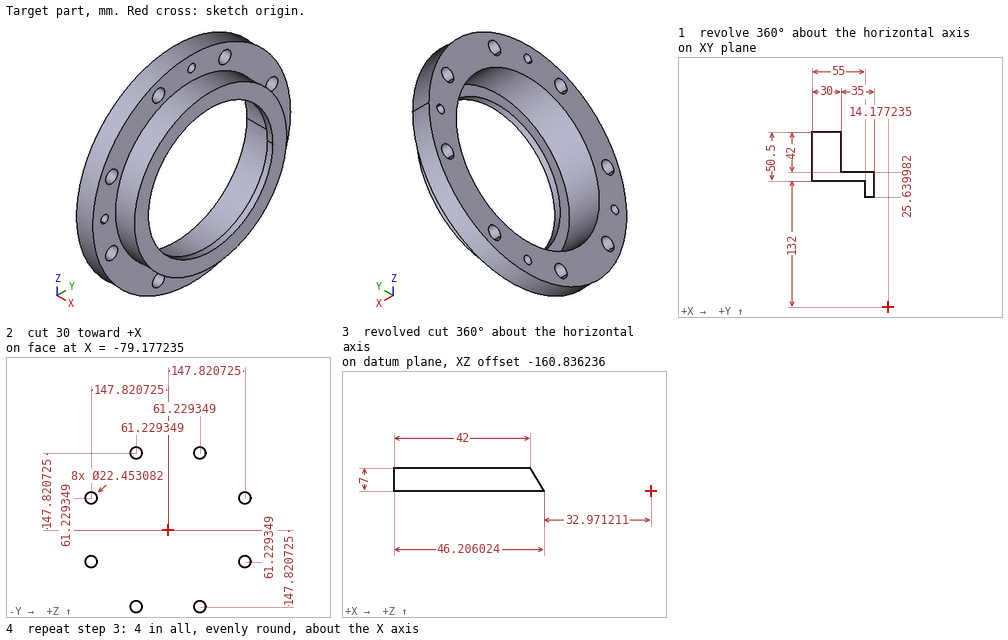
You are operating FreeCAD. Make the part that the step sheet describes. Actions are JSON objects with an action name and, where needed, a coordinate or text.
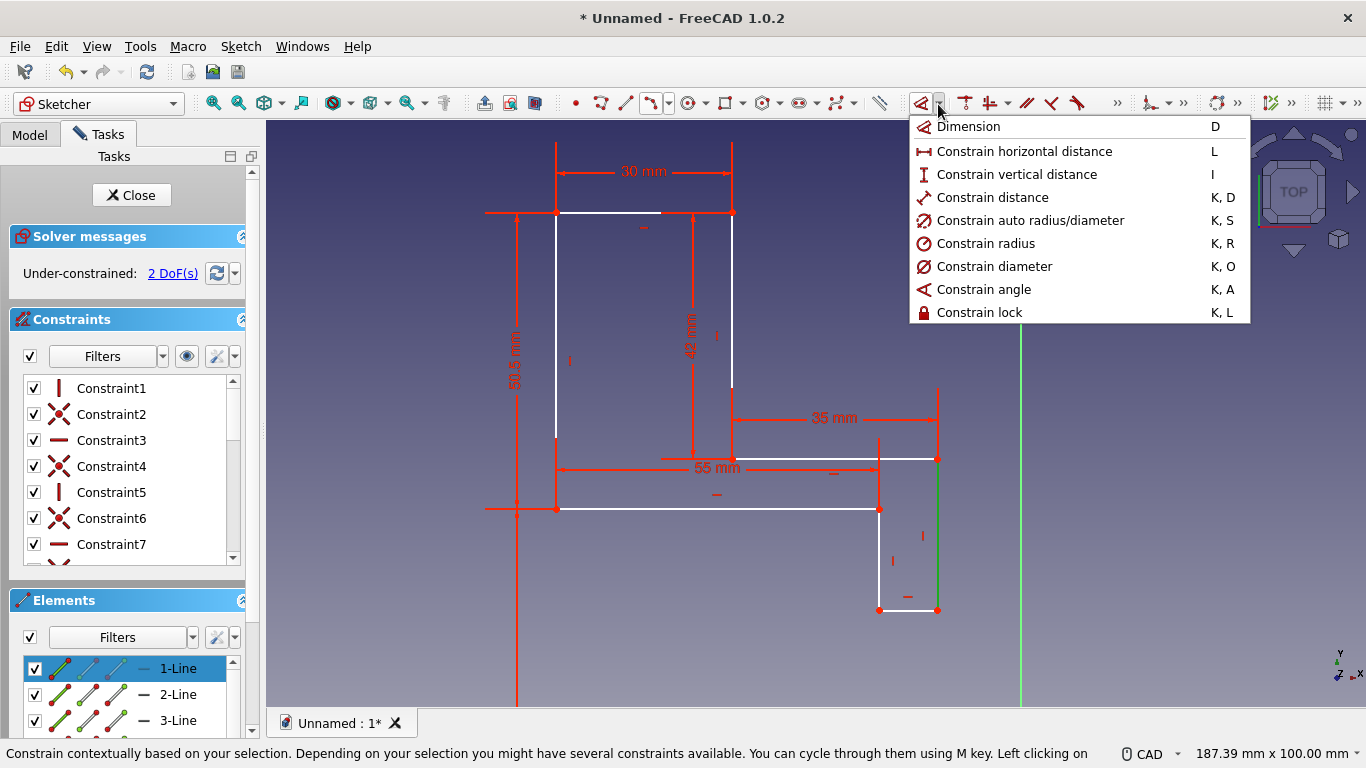
{"action": "left_click", "coordinate": [1080, 174]}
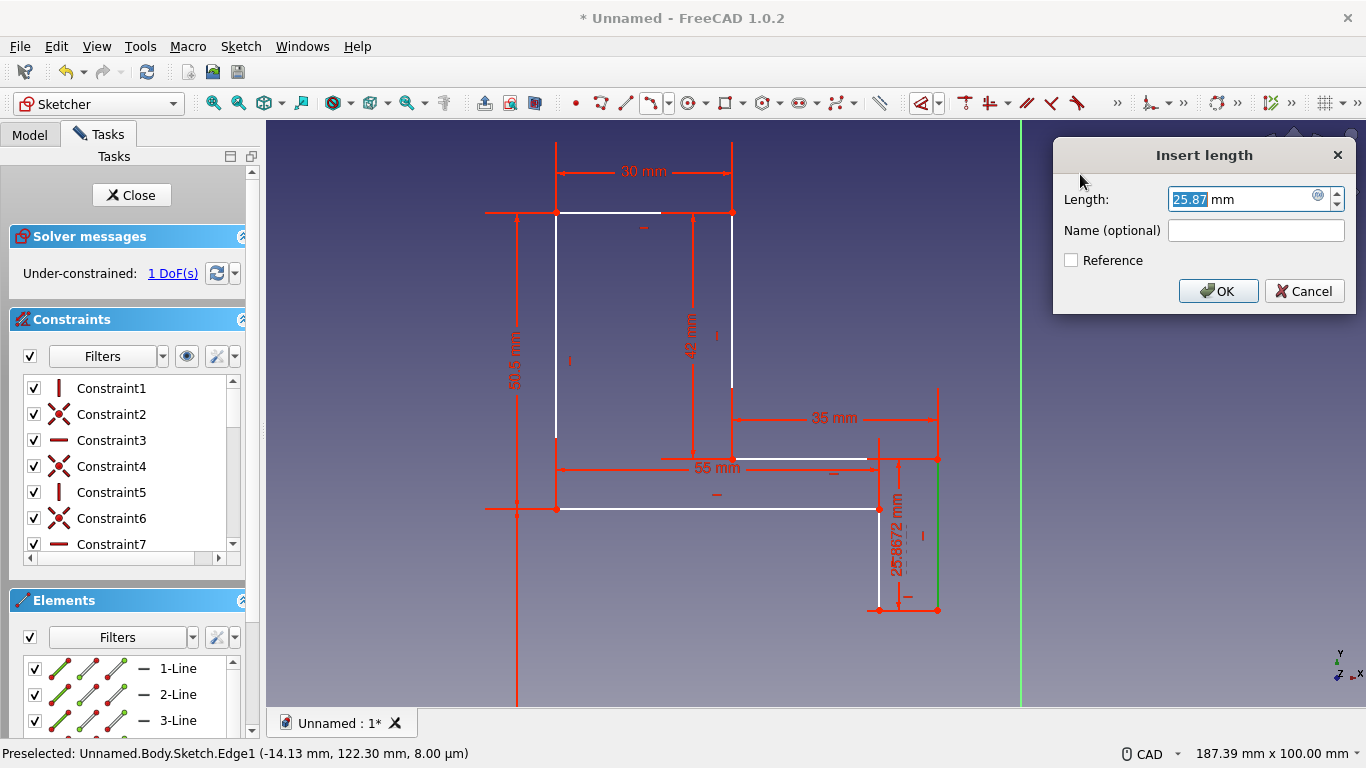
{"action": "type", "text": "25.639982"}
{"action": "key", "text": "Return"}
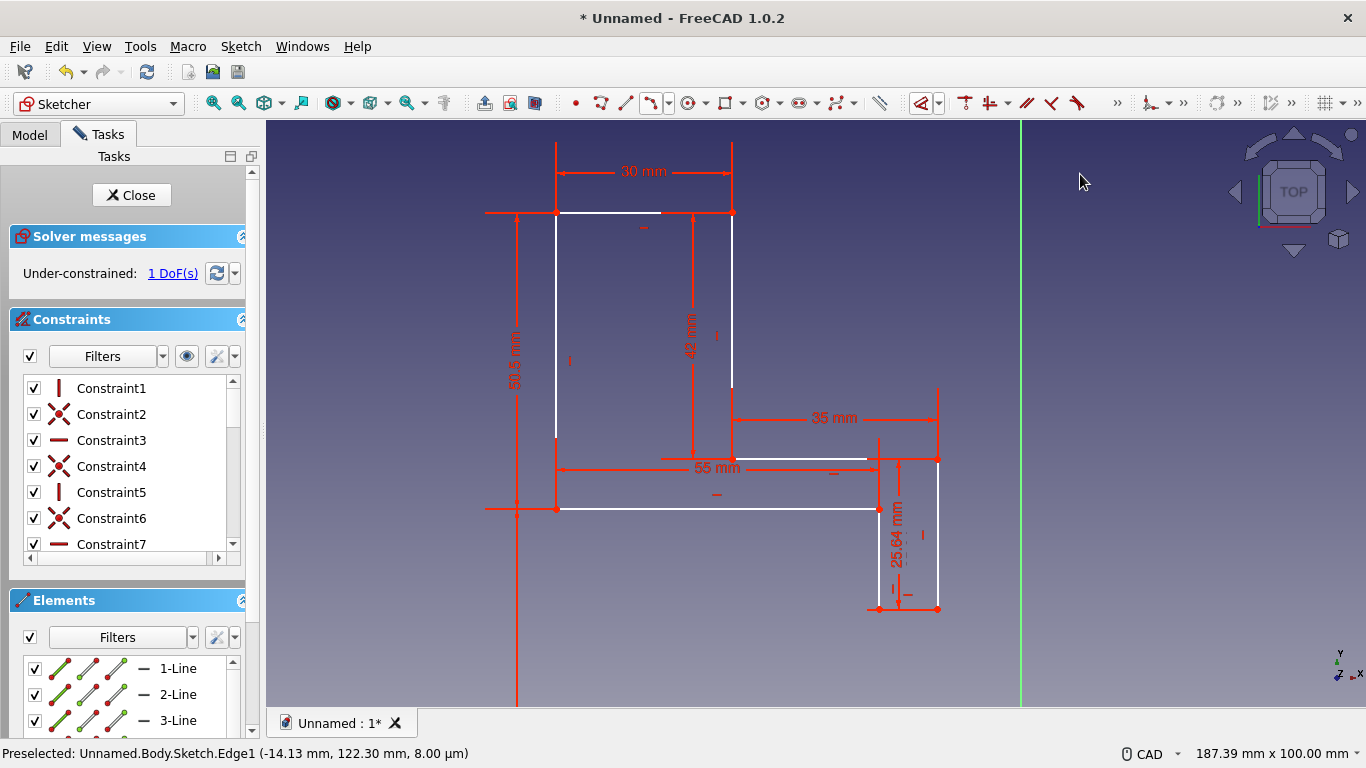
{"action": "left_click", "coordinate": [938, 610]}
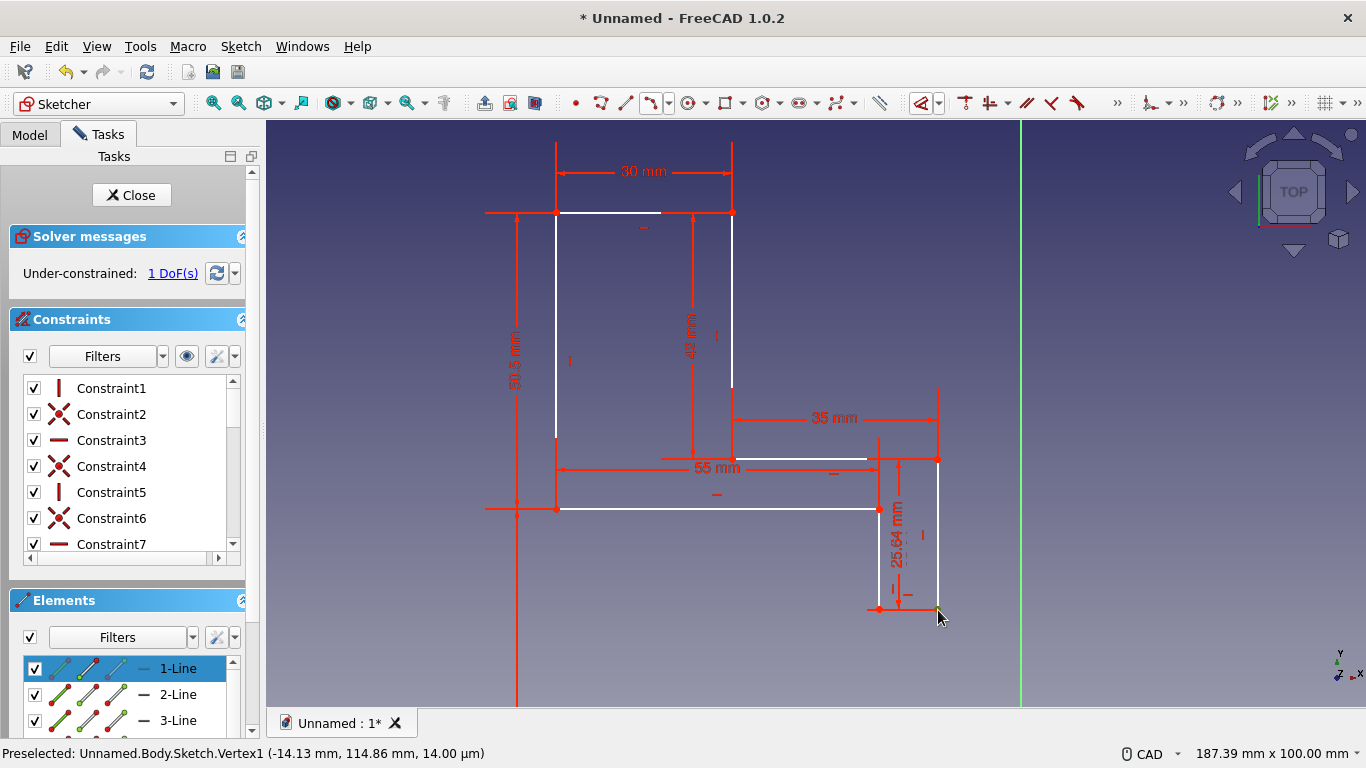
{"action": "left_click", "coordinate": [938, 104]}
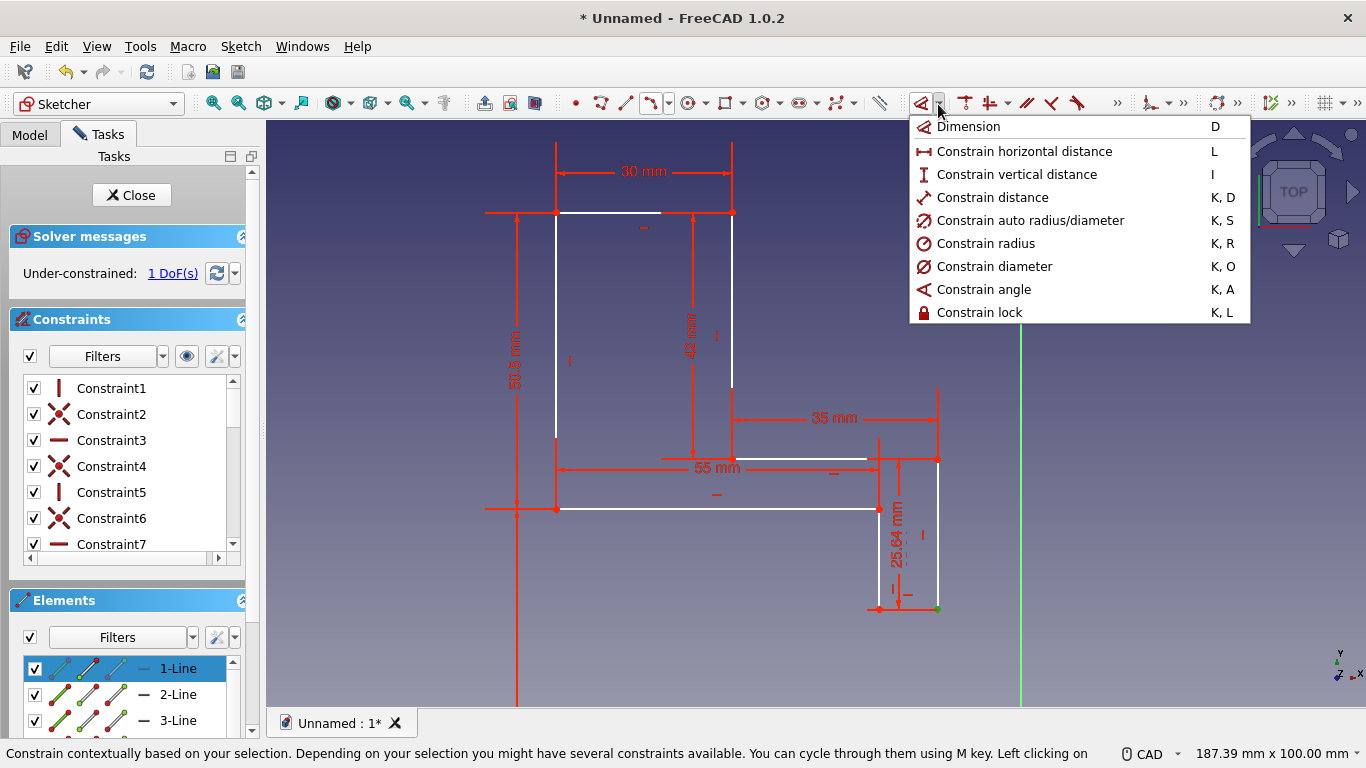
{"action": "left_click", "coordinate": [1080, 152]}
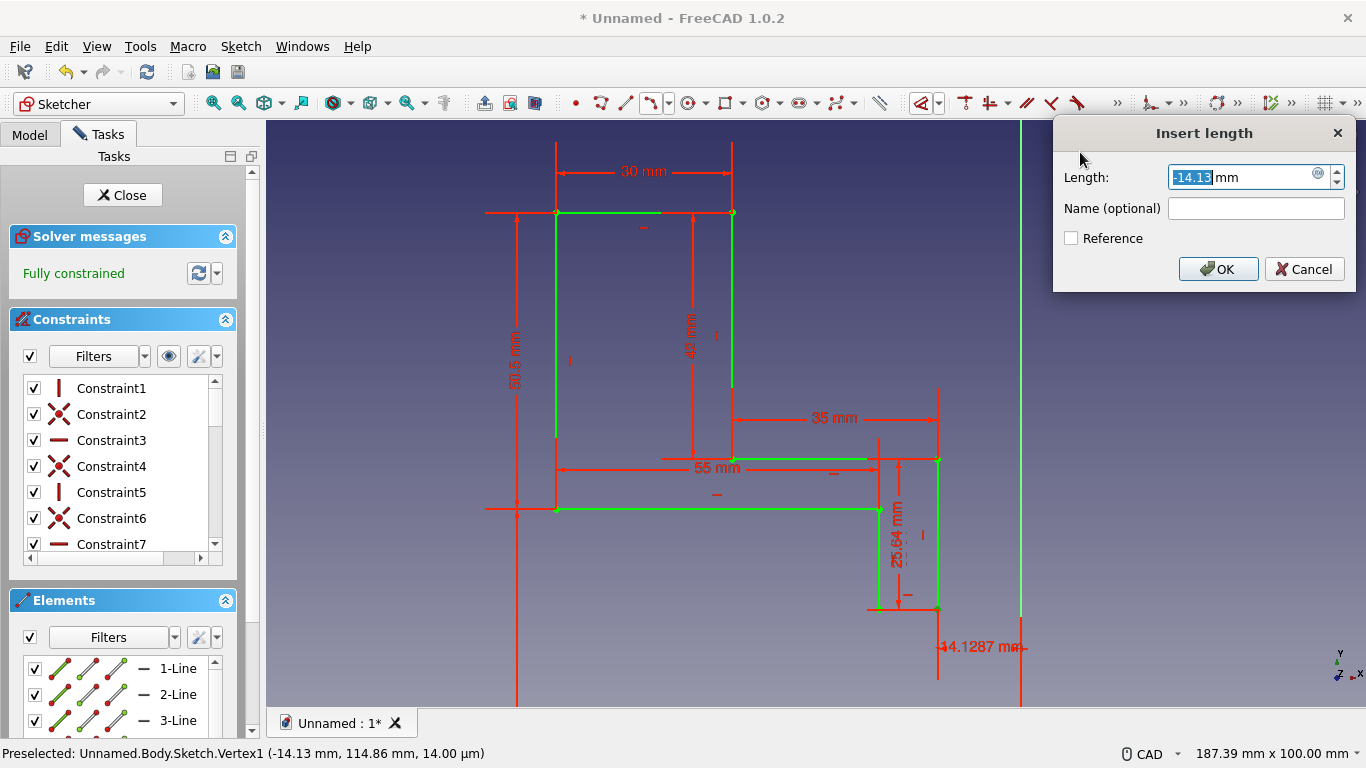
{"action": "type", "text": "-14.177235"}
{"action": "key", "text": "Return"}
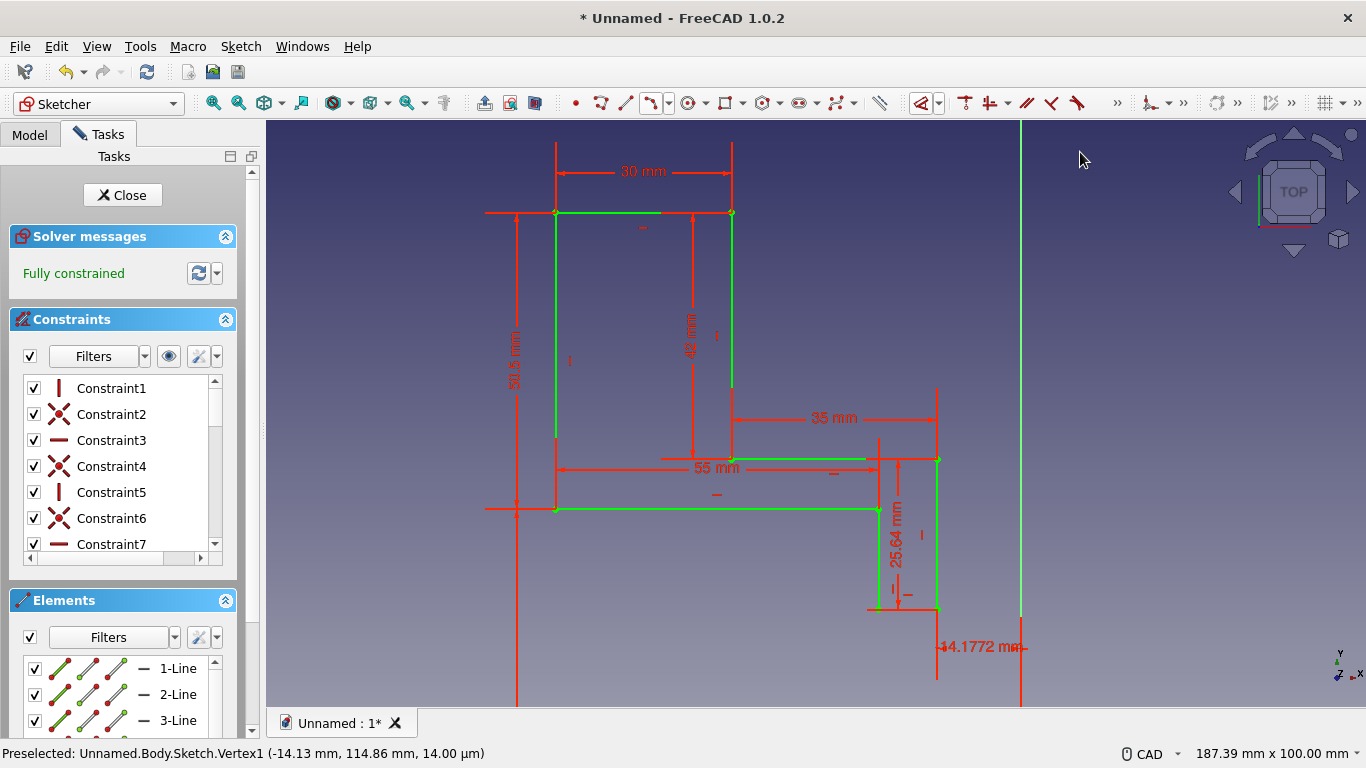
{"action": "left_click", "coordinate": [123, 195]}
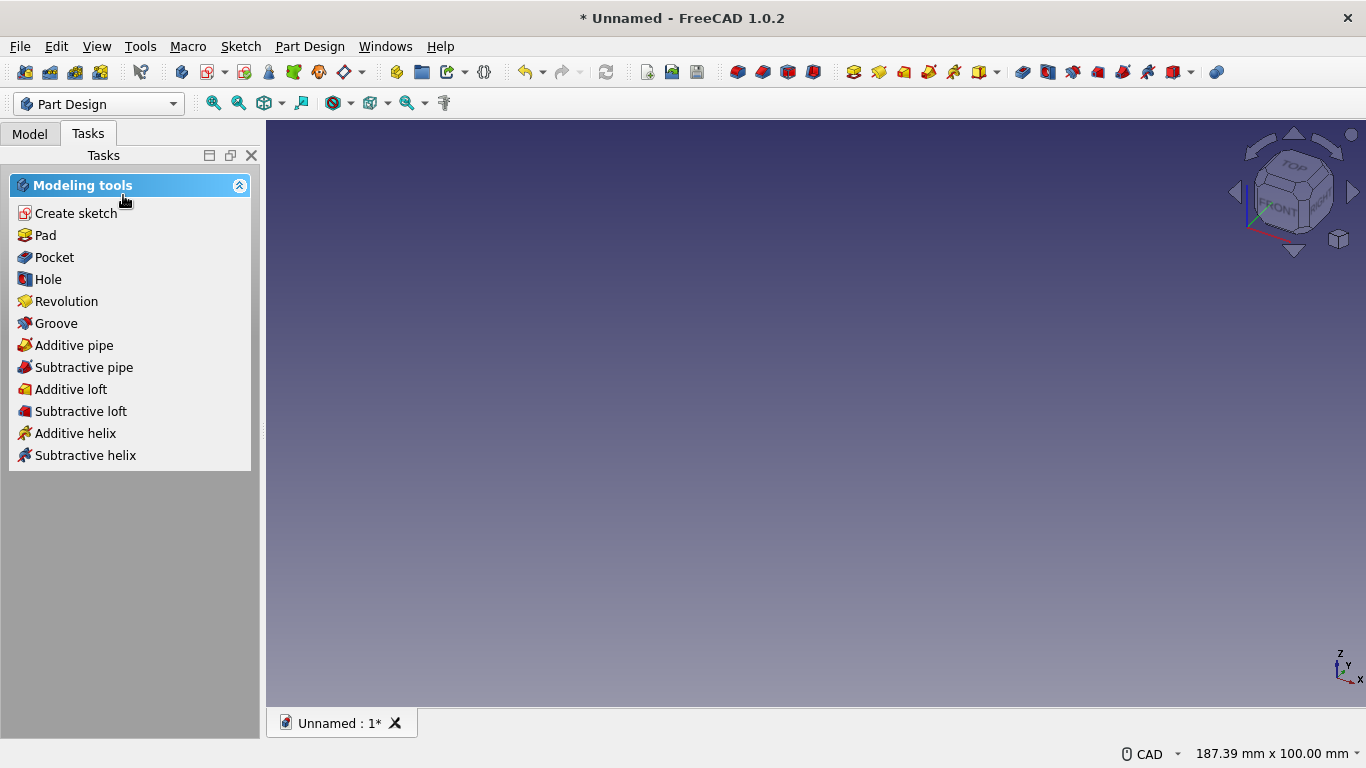
{"action": "left_click", "coordinate": [879, 72]}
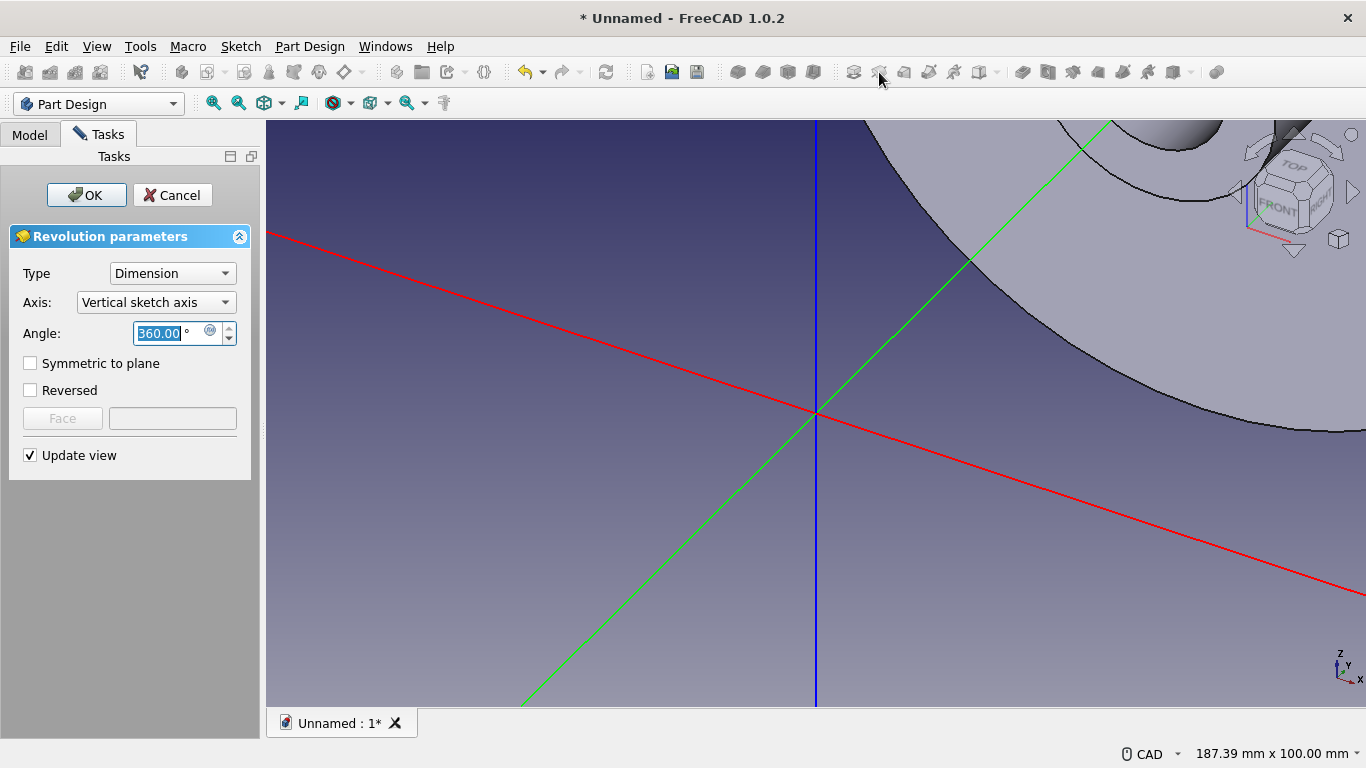
{"action": "left_click", "coordinate": [157, 302]}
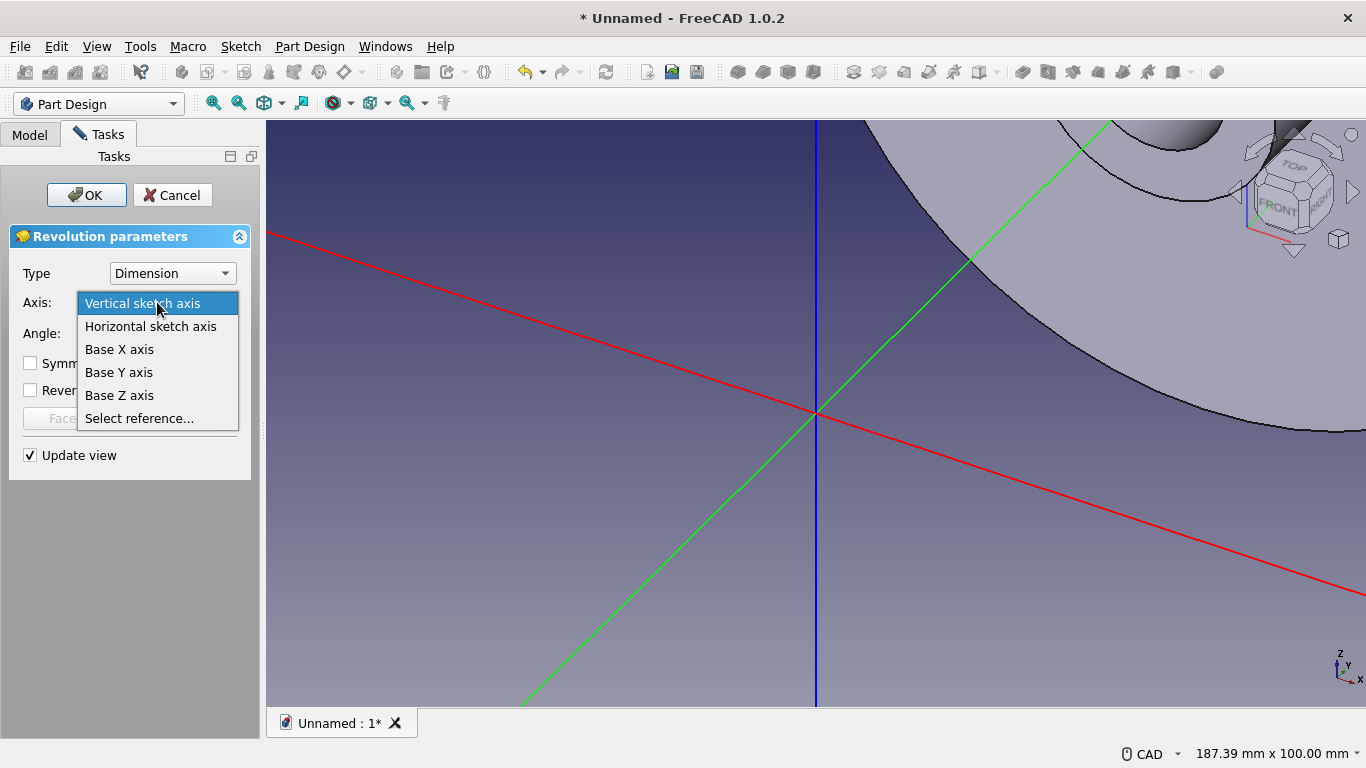
{"action": "left_click", "coordinate": [156, 326]}